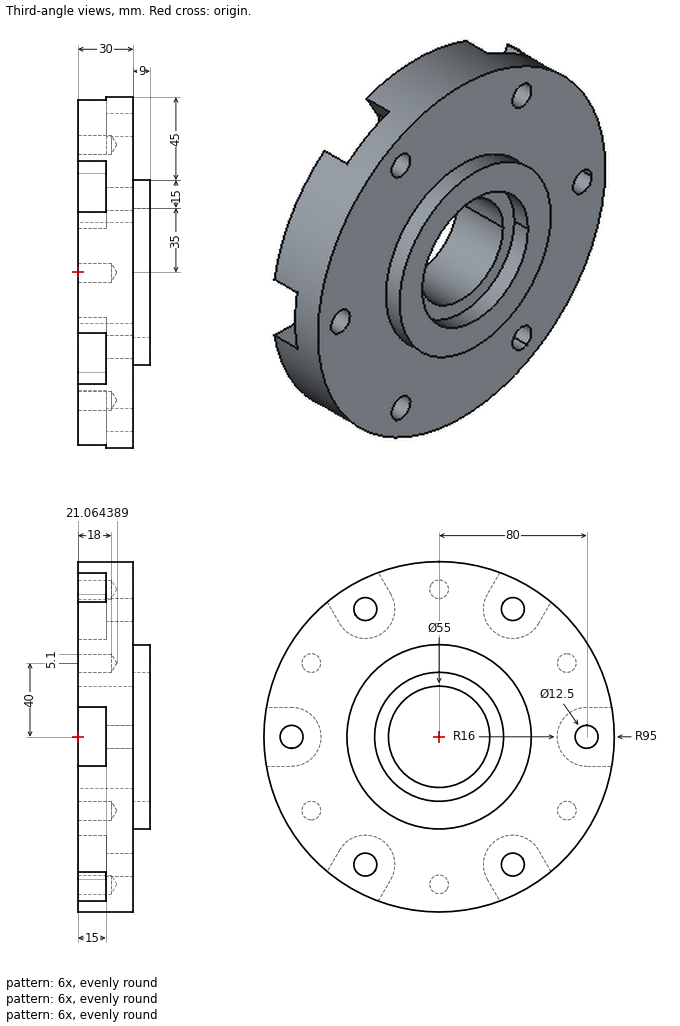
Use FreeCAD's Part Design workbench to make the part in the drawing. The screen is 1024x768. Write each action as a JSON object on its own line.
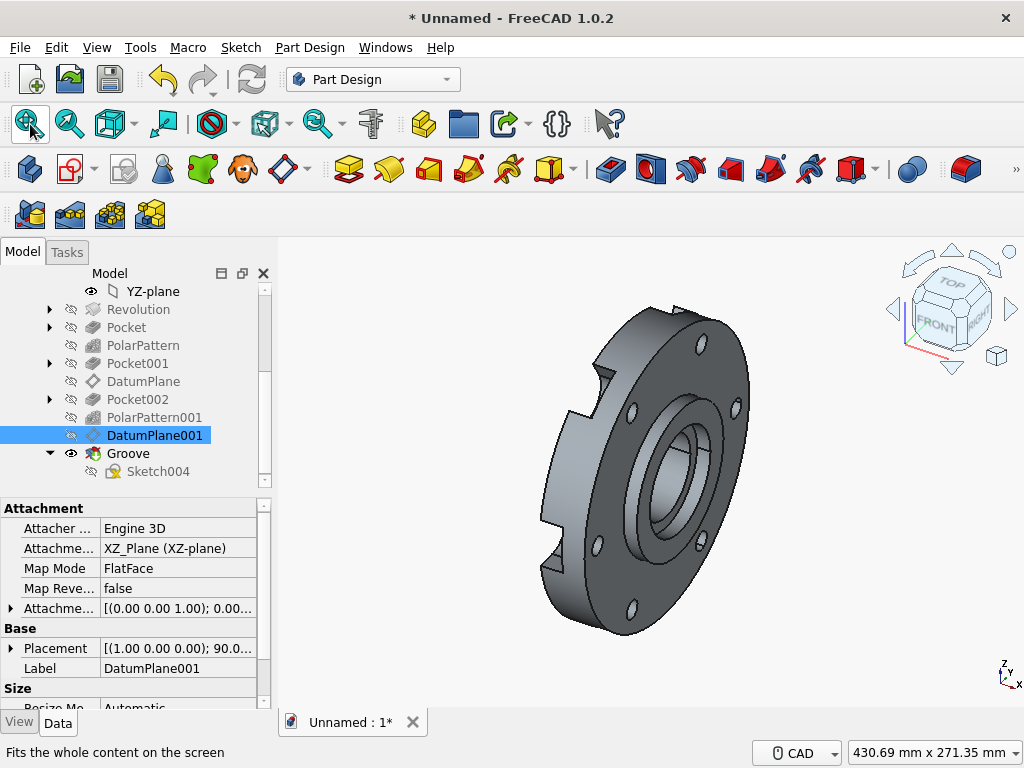
{"action": "left_click", "coordinate": [116, 453]}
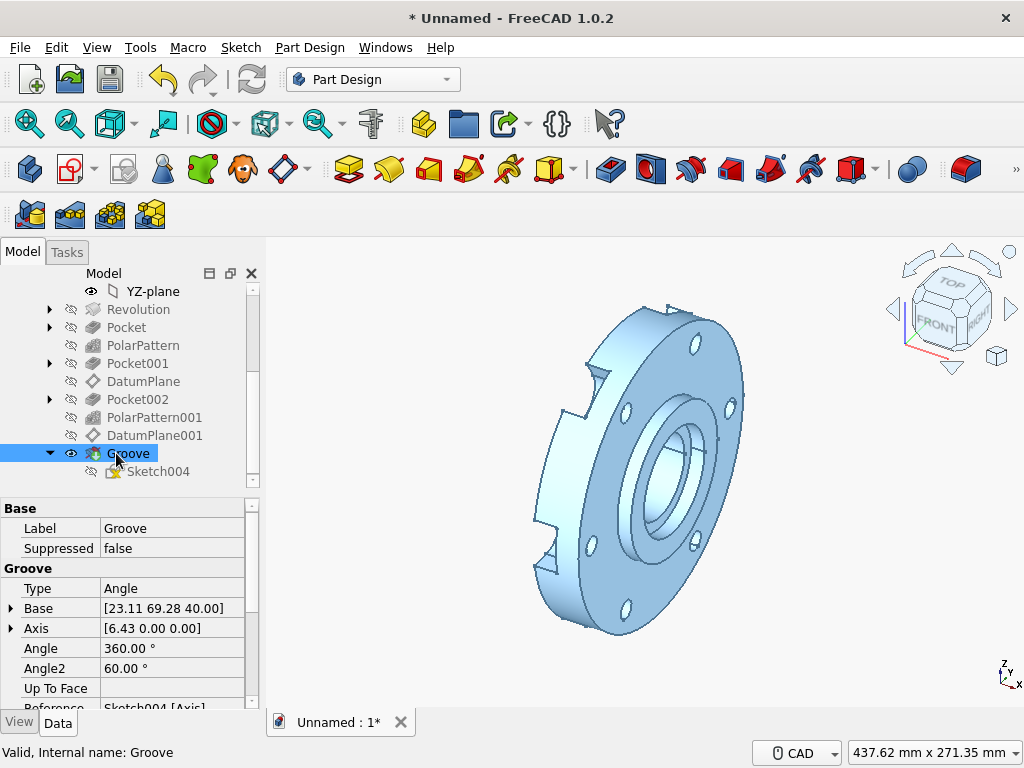
{"action": "left_click", "coordinate": [110, 214]}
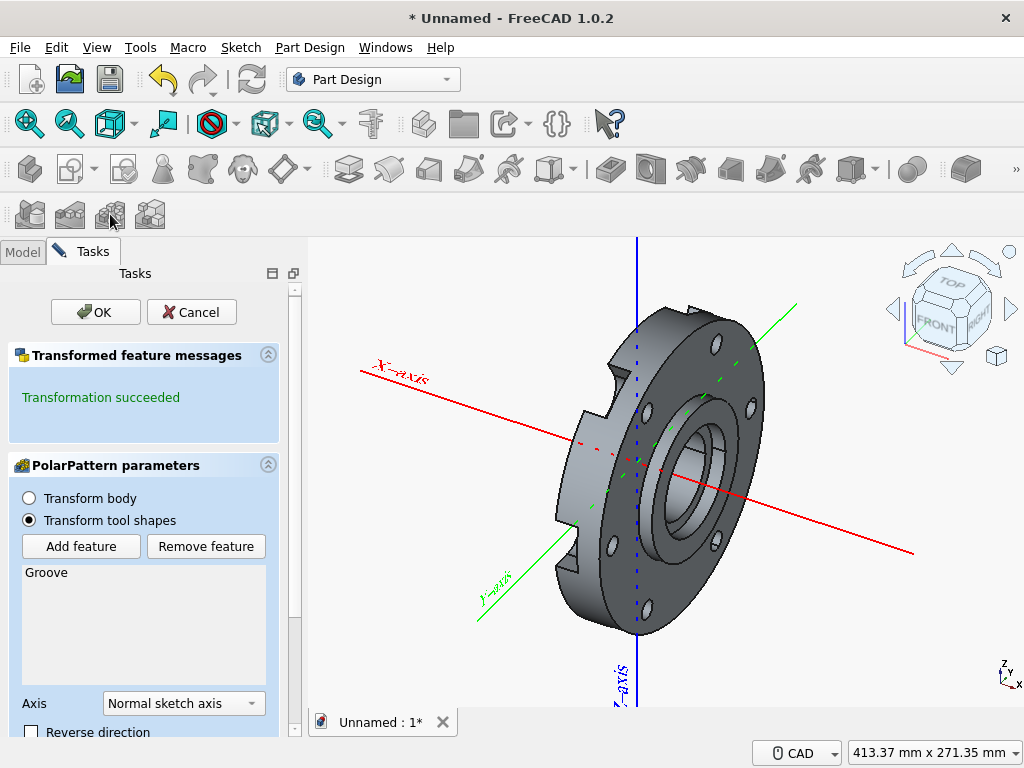
{"action": "left_click", "coordinate": [184, 704]}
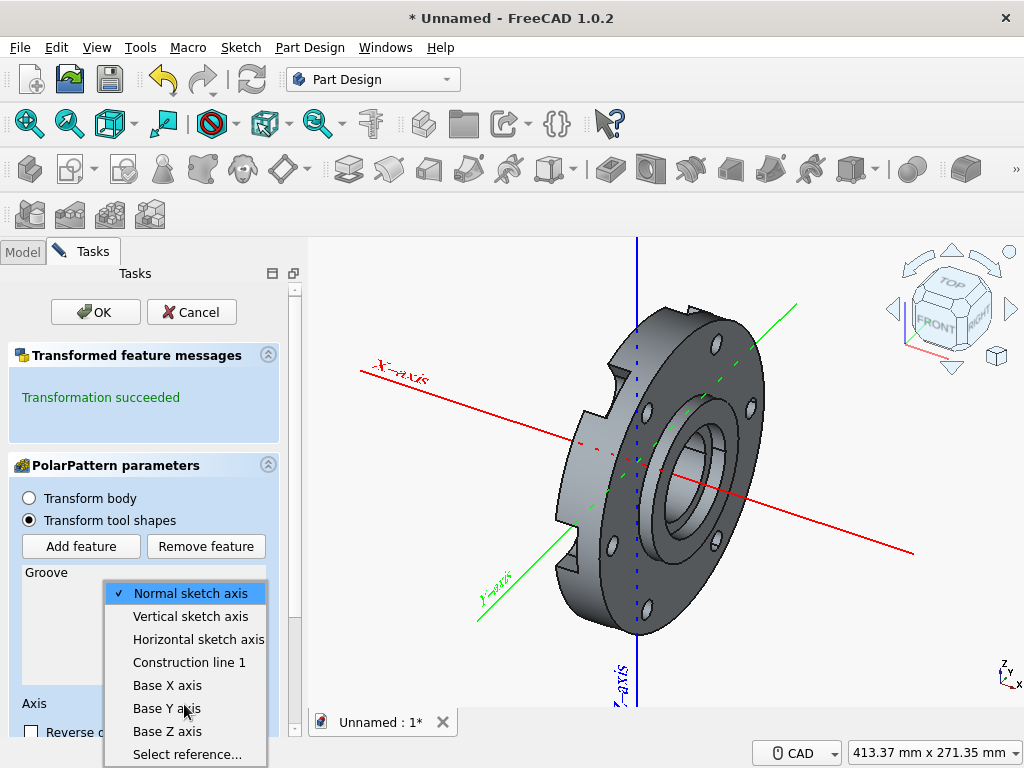
{"action": "left_click", "coordinate": [184, 686]}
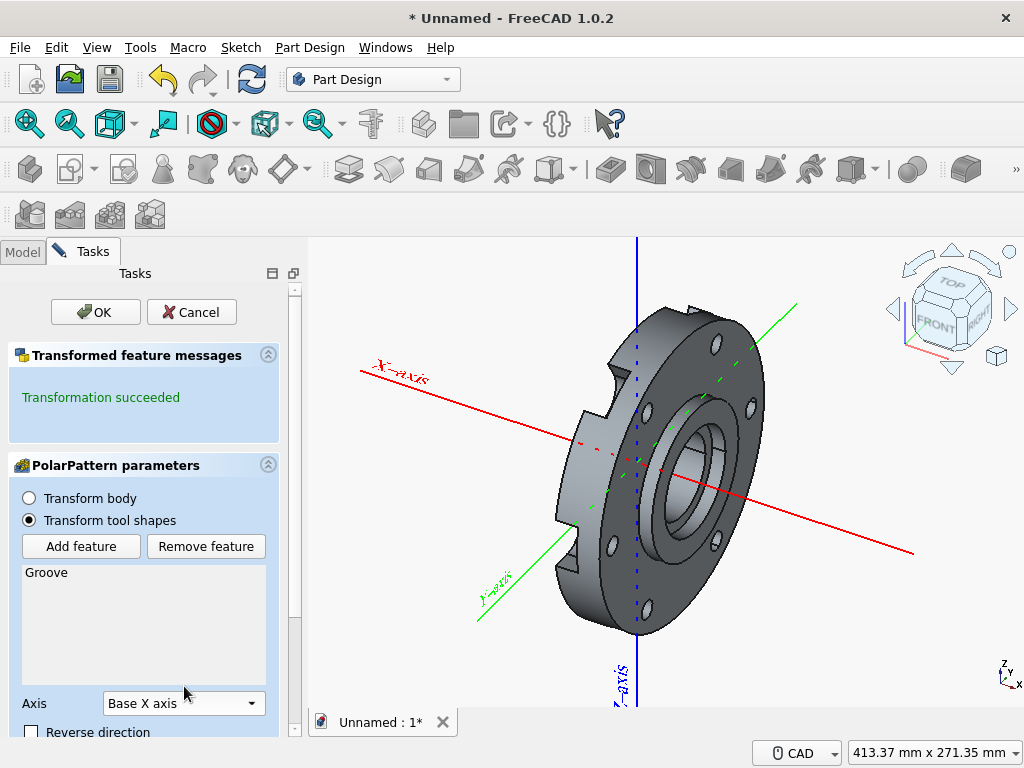
{"action": "scroll", "coordinate": [295, 510], "scroll_direction": "down", "scroll_amount": 3}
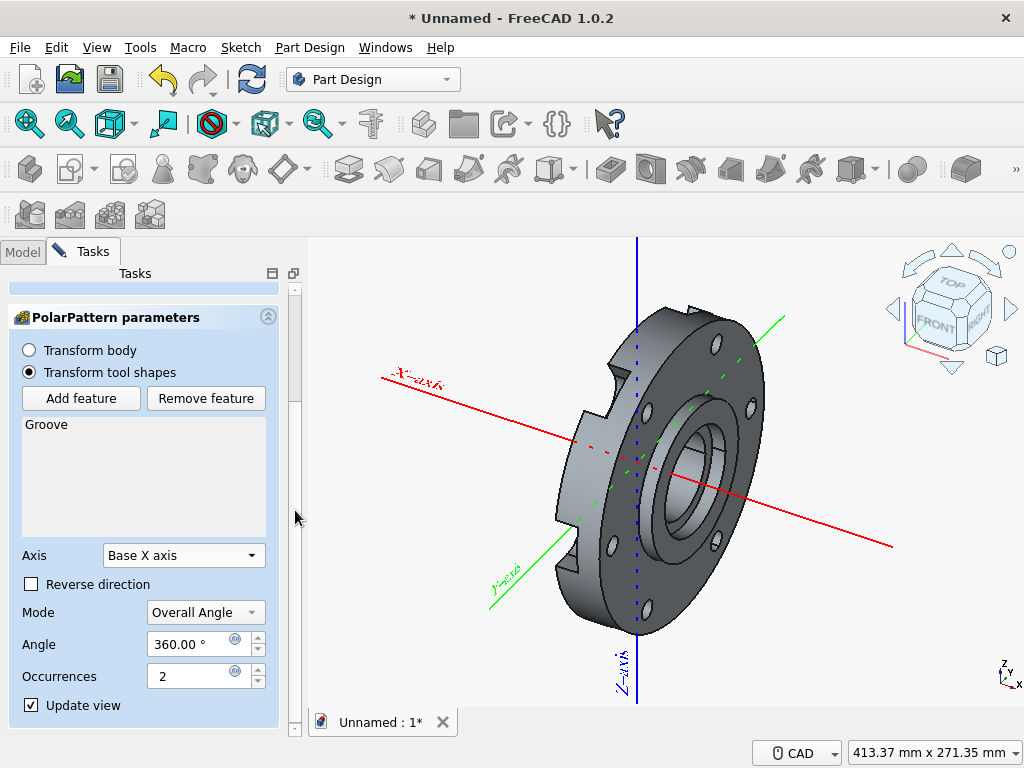
{"action": "triple_click", "coordinate": [198, 676]}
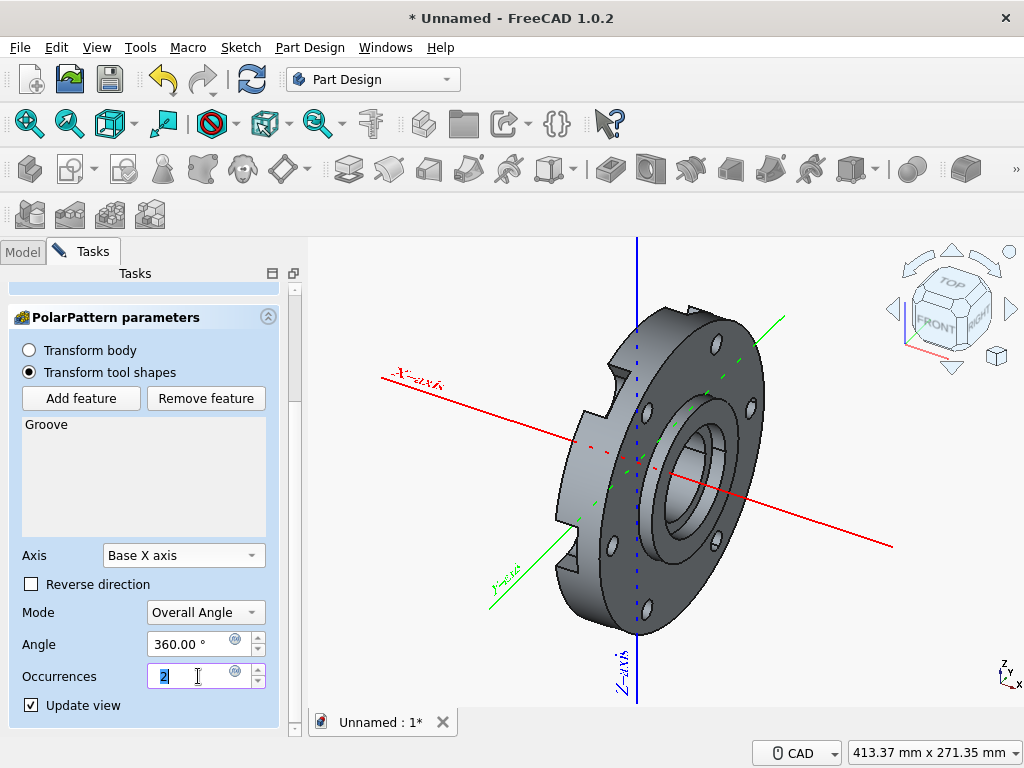
{"action": "type", "text": "6"}
{"action": "key", "text": "Tab"}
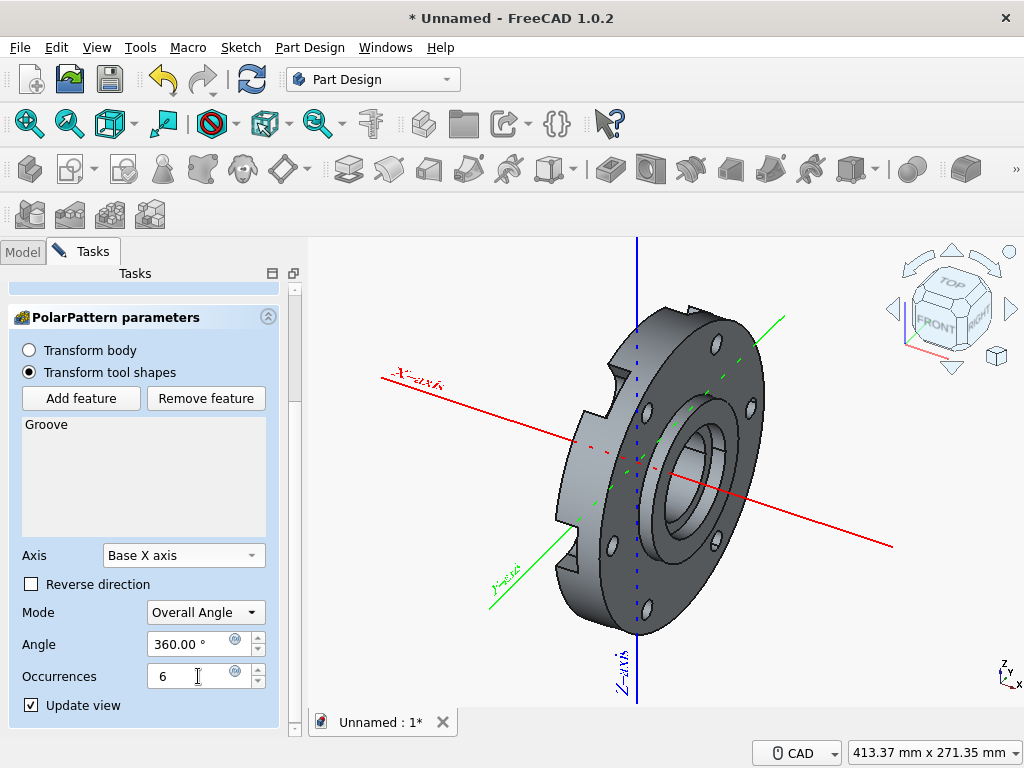
{"action": "scroll", "coordinate": [295, 510], "scroll_direction": "up", "scroll_amount": 4}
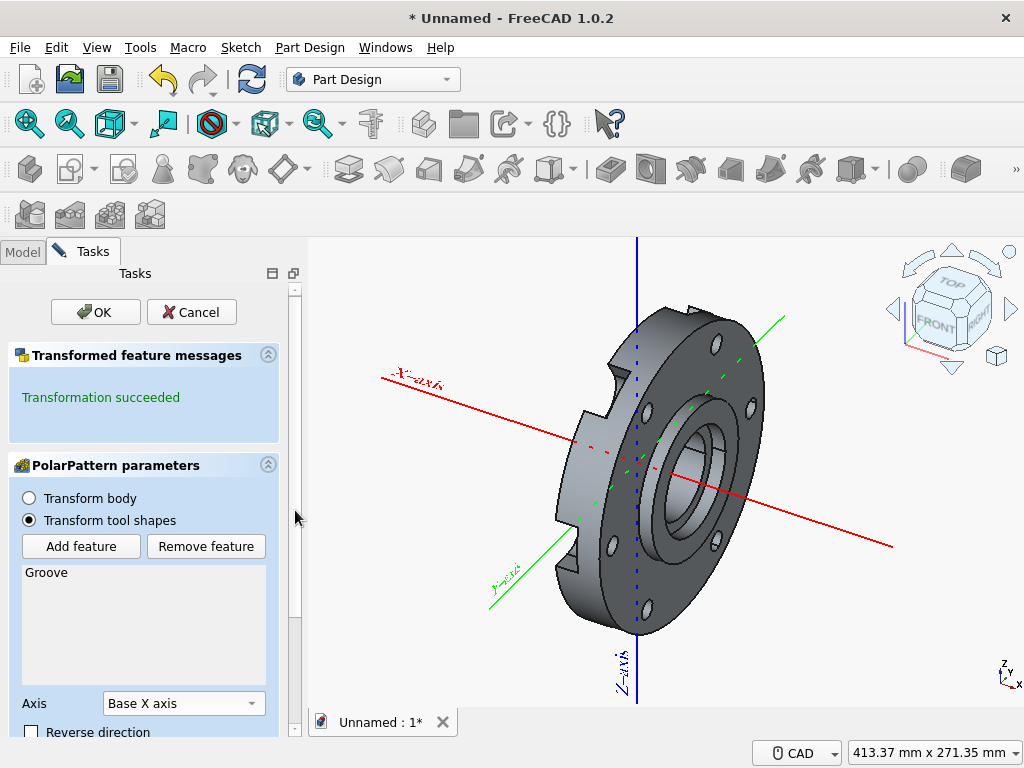
{"action": "left_click", "coordinate": [96, 312]}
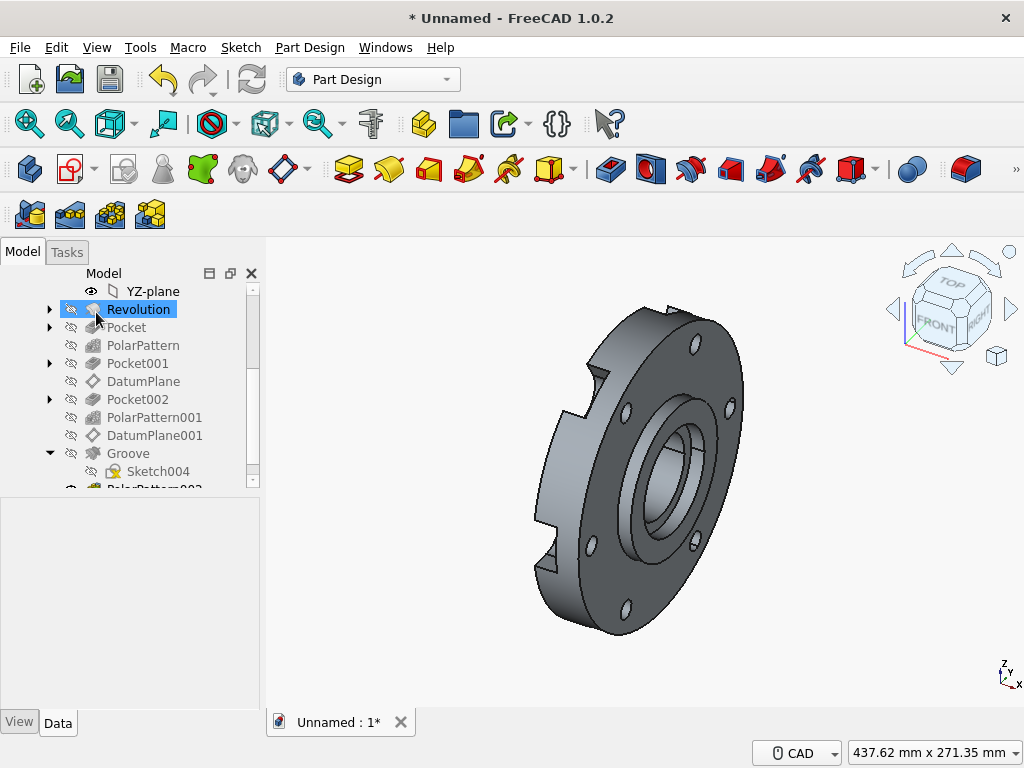
{"action": "key", "text": "0"}